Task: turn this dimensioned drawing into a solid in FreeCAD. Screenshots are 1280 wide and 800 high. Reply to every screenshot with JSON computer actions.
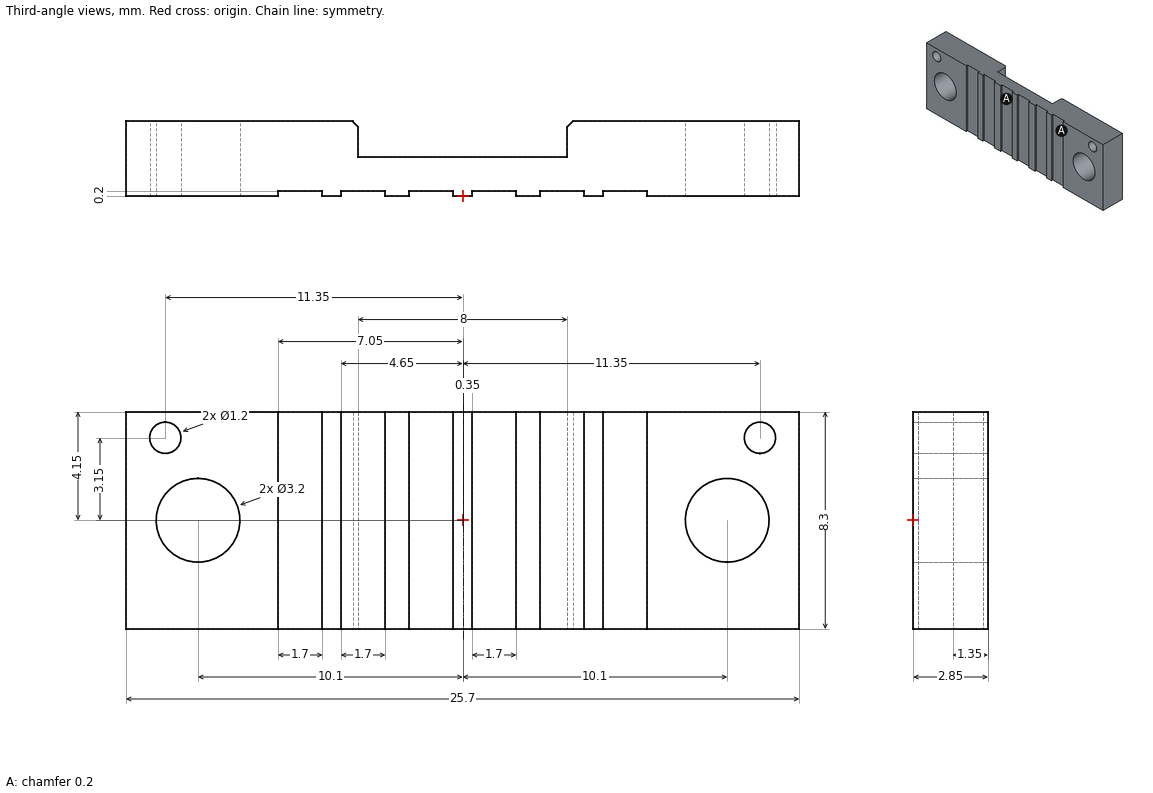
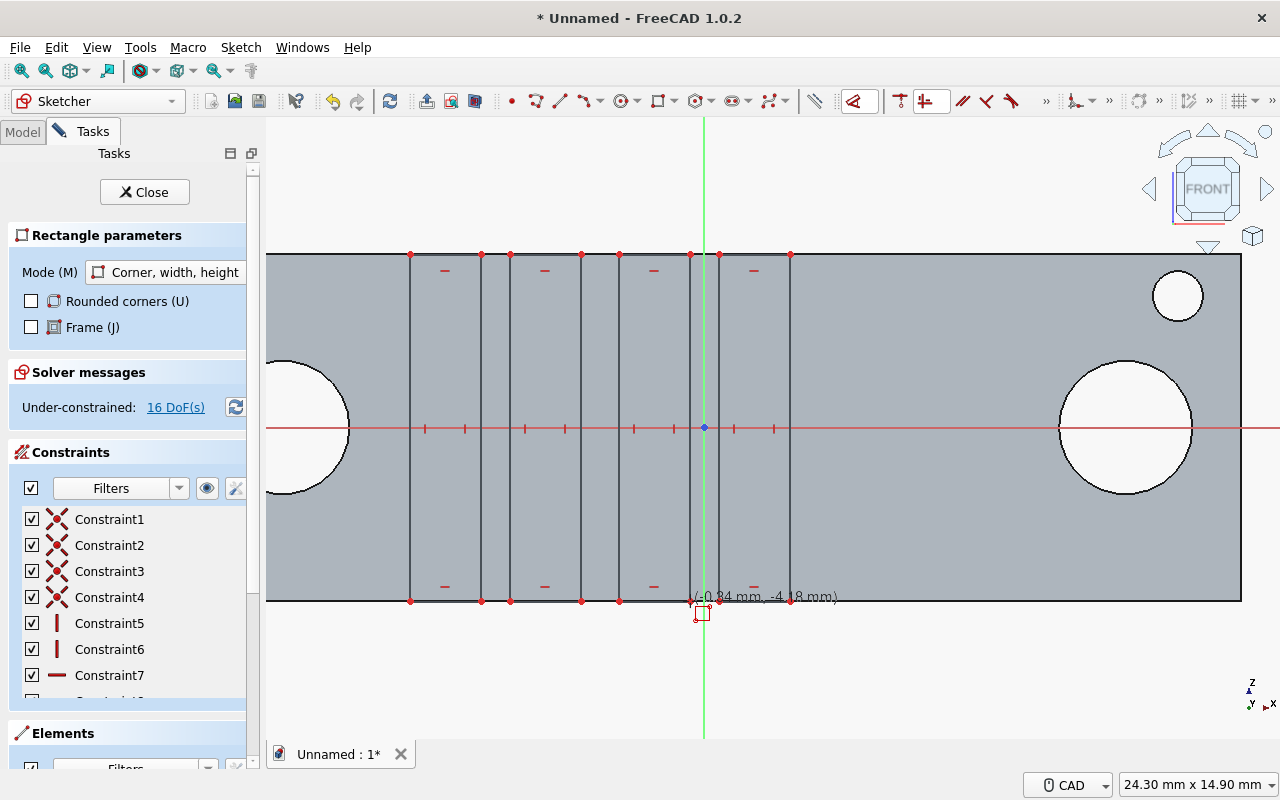
{"action": "left_click", "coordinate": [827, 254]}
{"action": "left_click", "coordinate": [898, 601]}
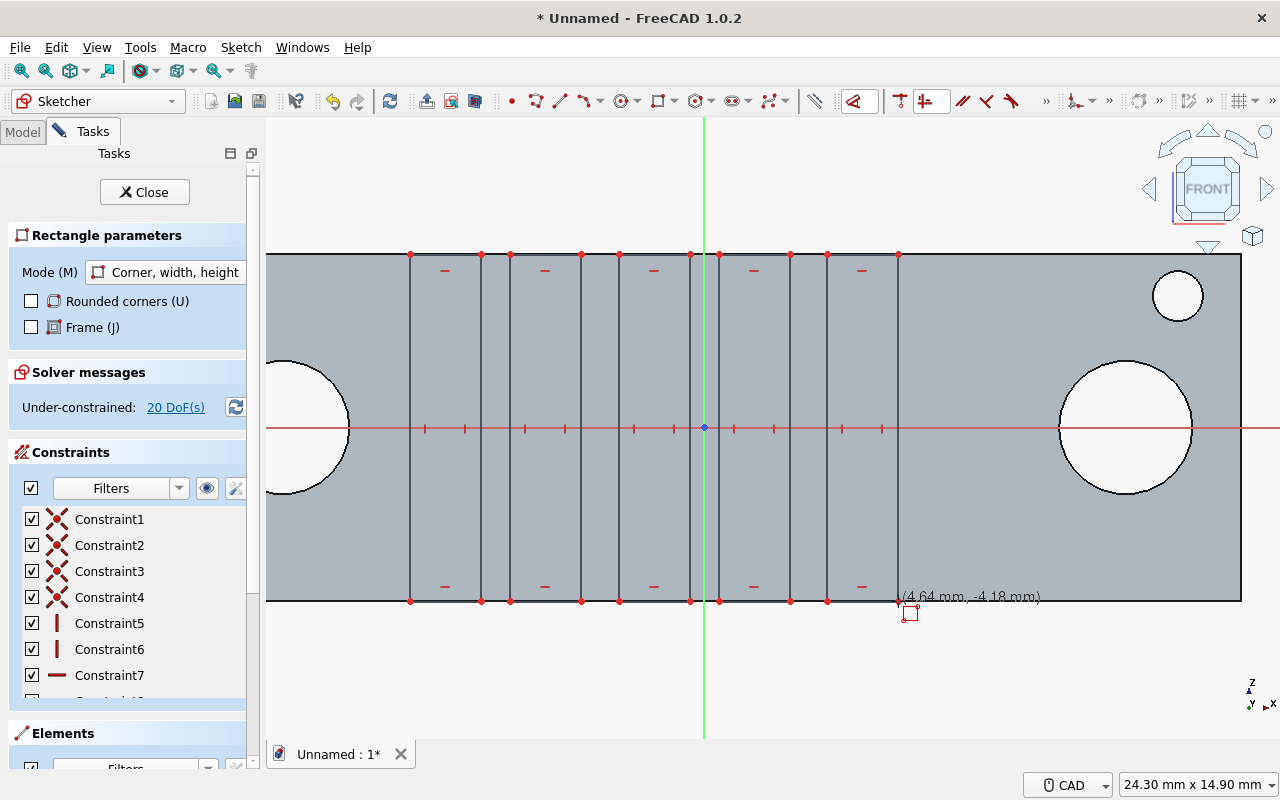
{"action": "left_click", "coordinate": [928, 254]}
{"action": "left_click", "coordinate": [999, 601]}
{"action": "key", "text": "Escape"}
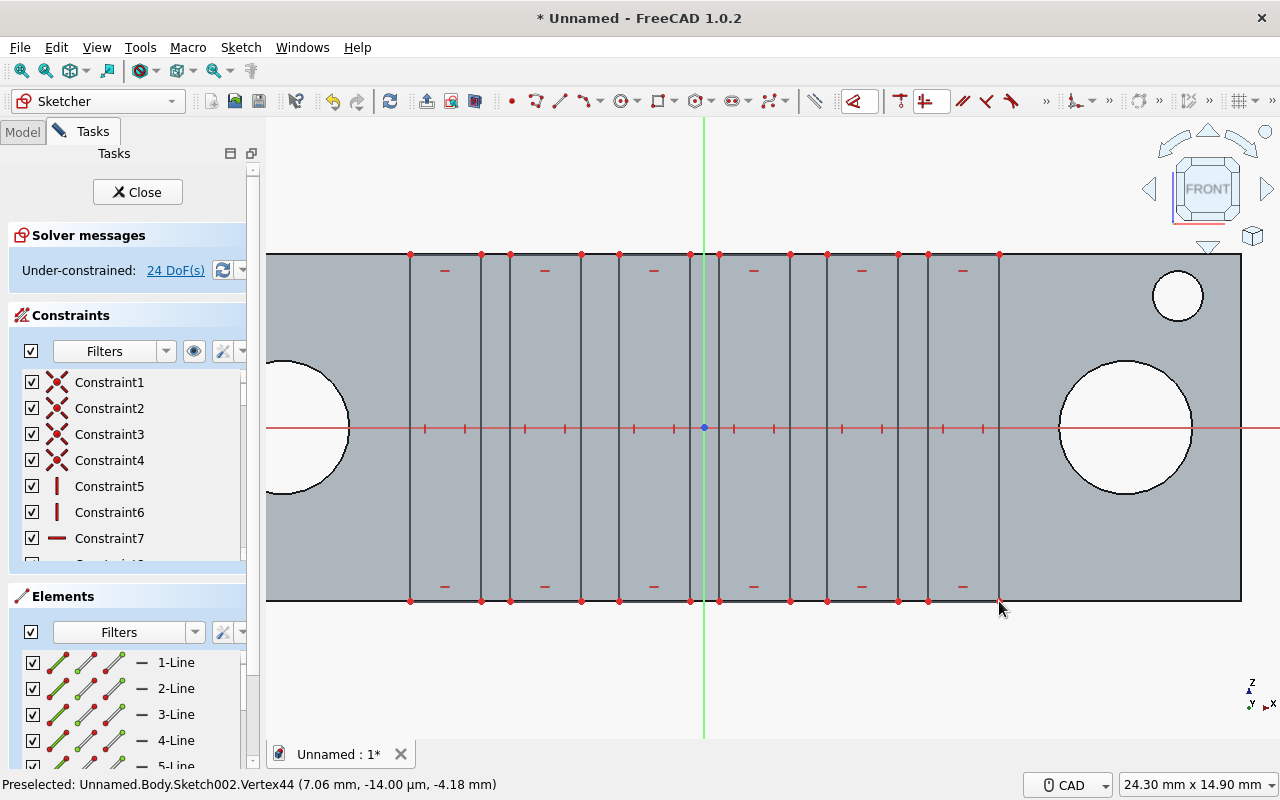
{"action": "left_click", "coordinate": [790, 255]}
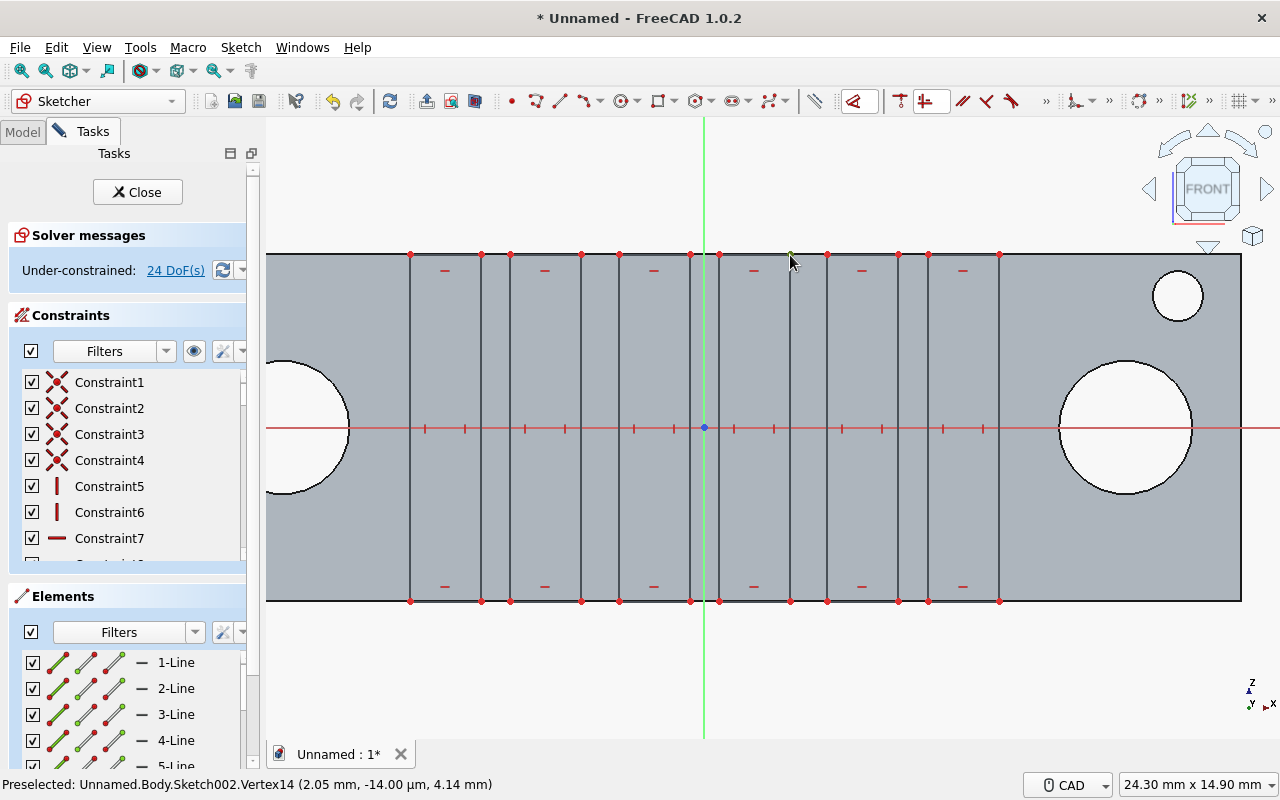
{"action": "left_click", "coordinate": [619, 255]}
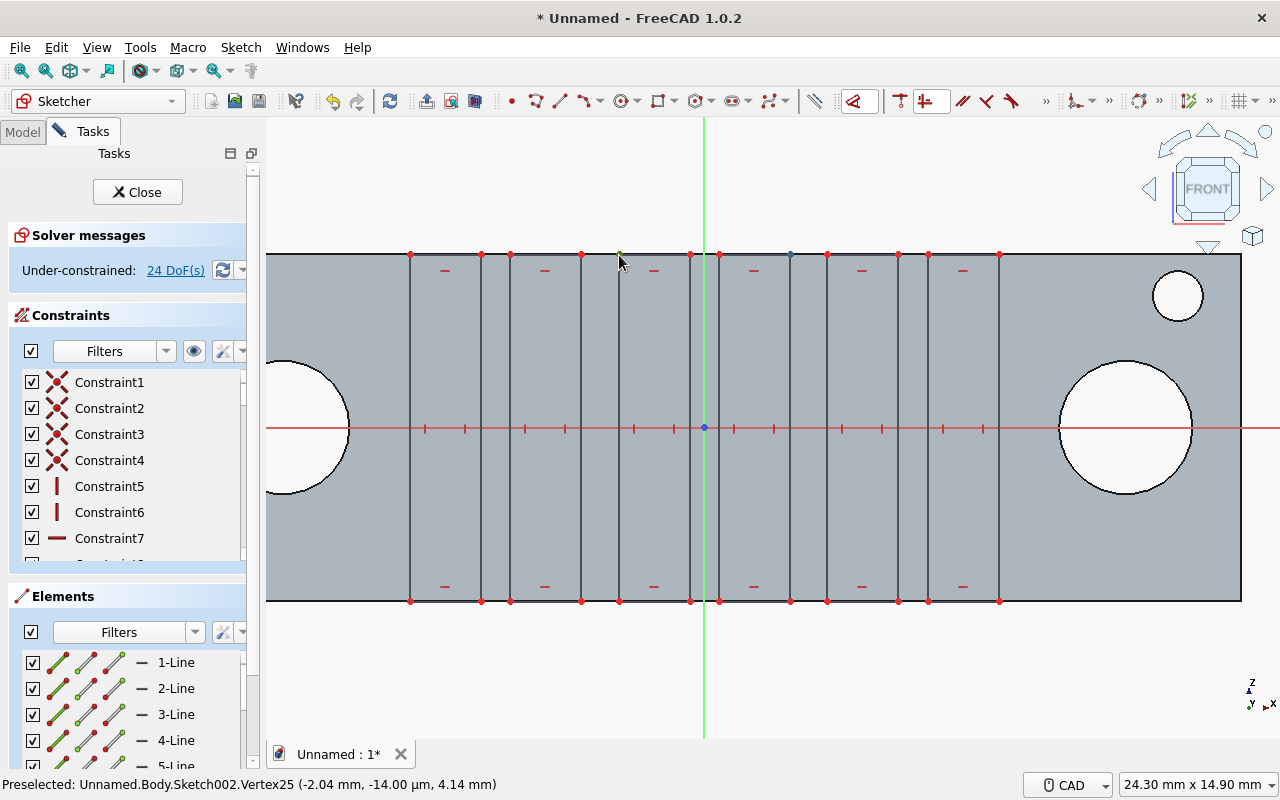
{"action": "left_click", "coordinate": [704, 671]}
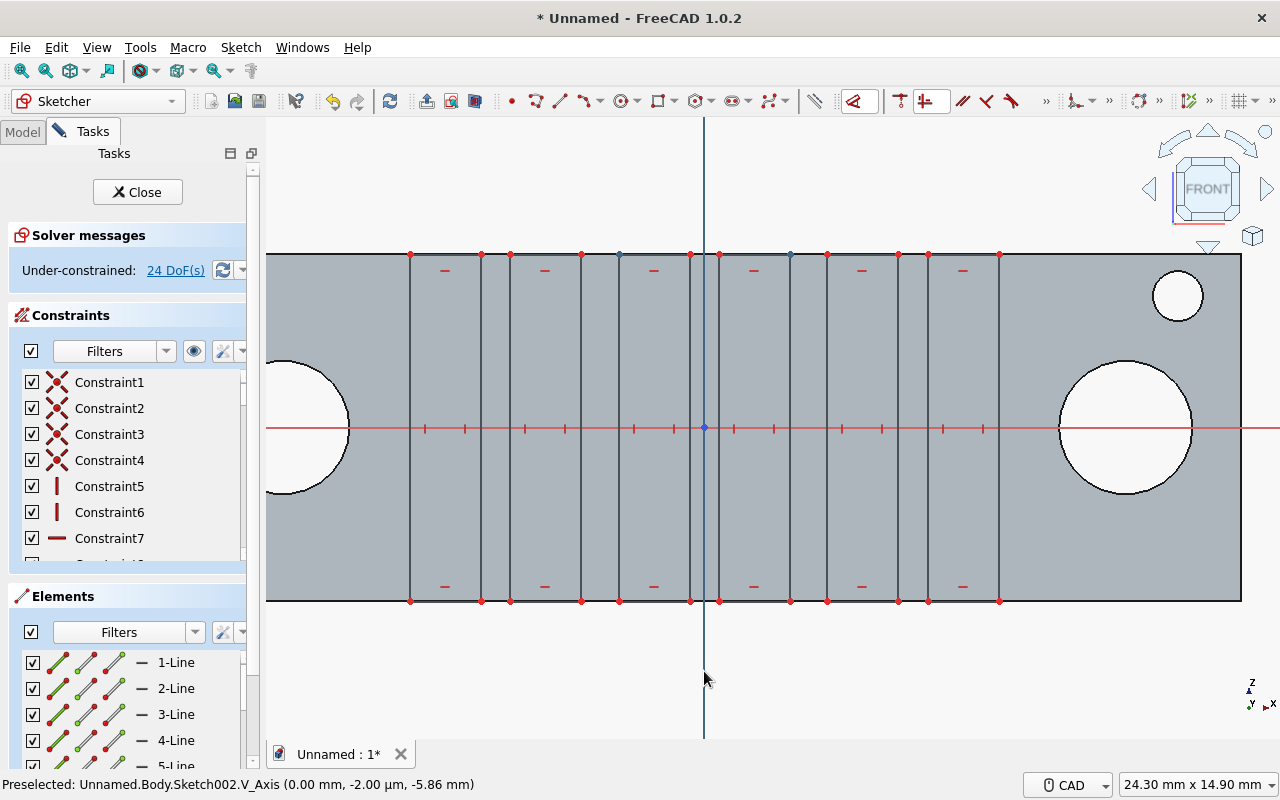
{"action": "key", "text": "s"}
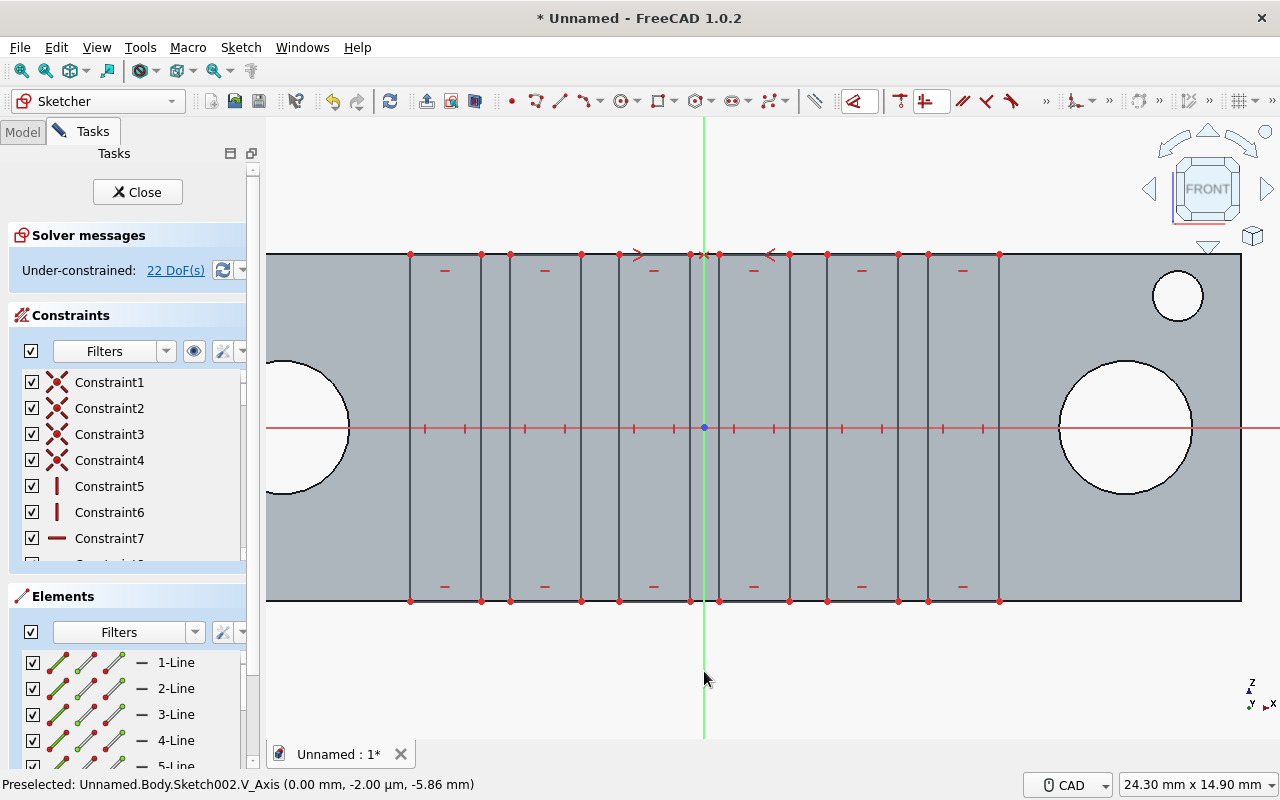
{"action": "left_click", "coordinate": [719, 602]}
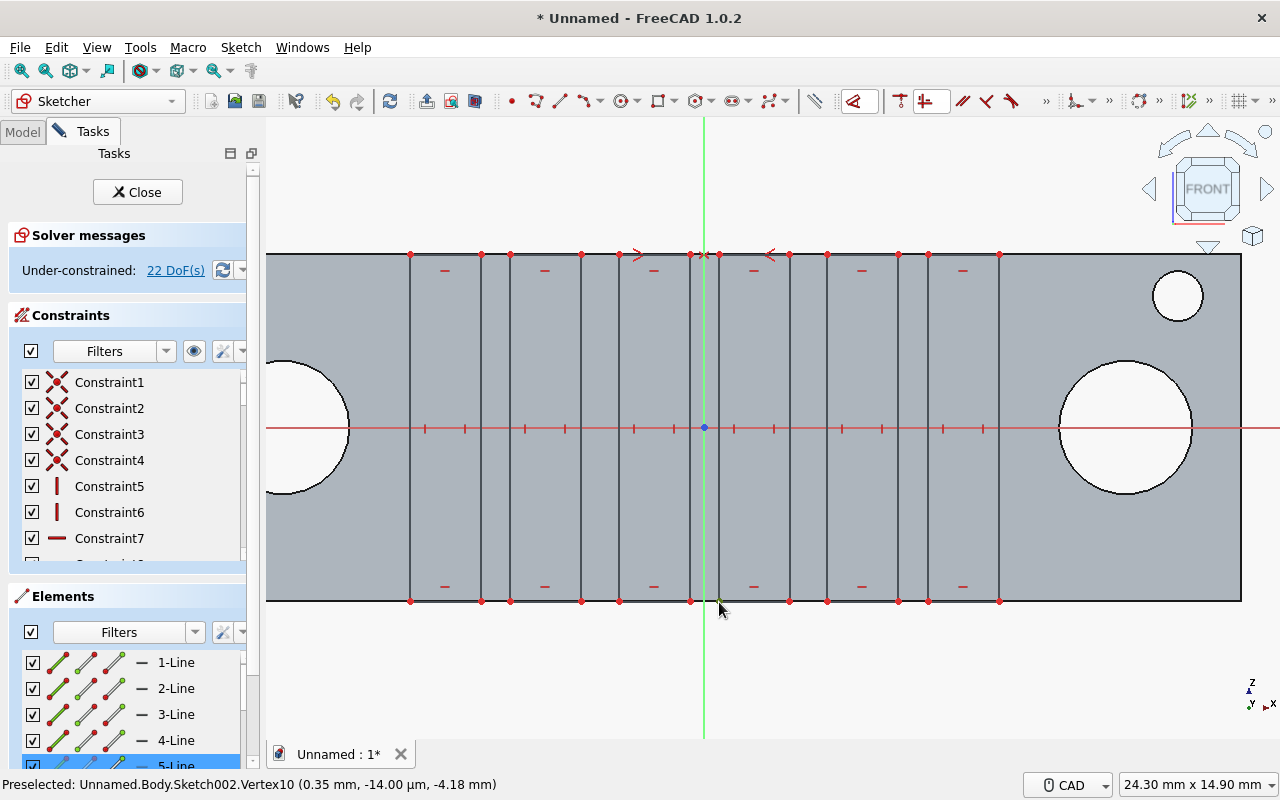
{"action": "left_click", "coordinate": [690, 602]}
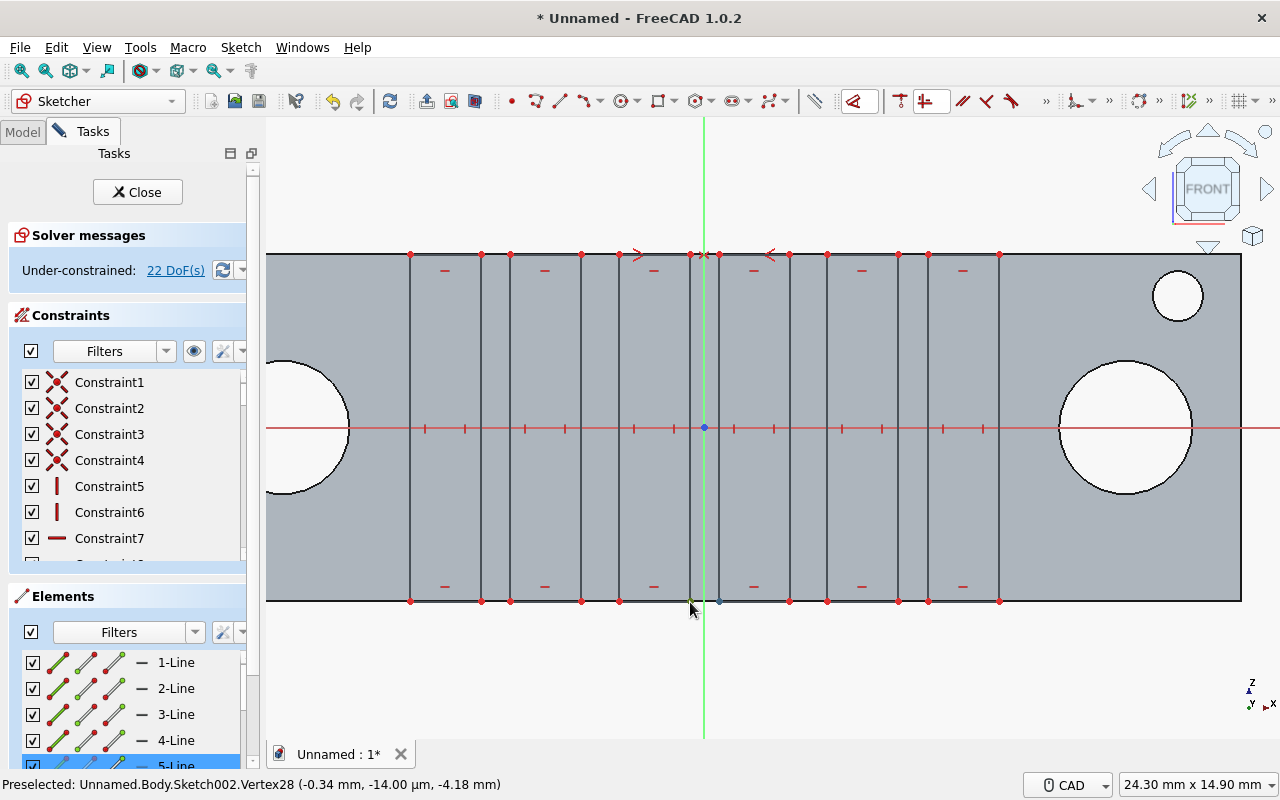
{"action": "left_click", "coordinate": [704, 671]}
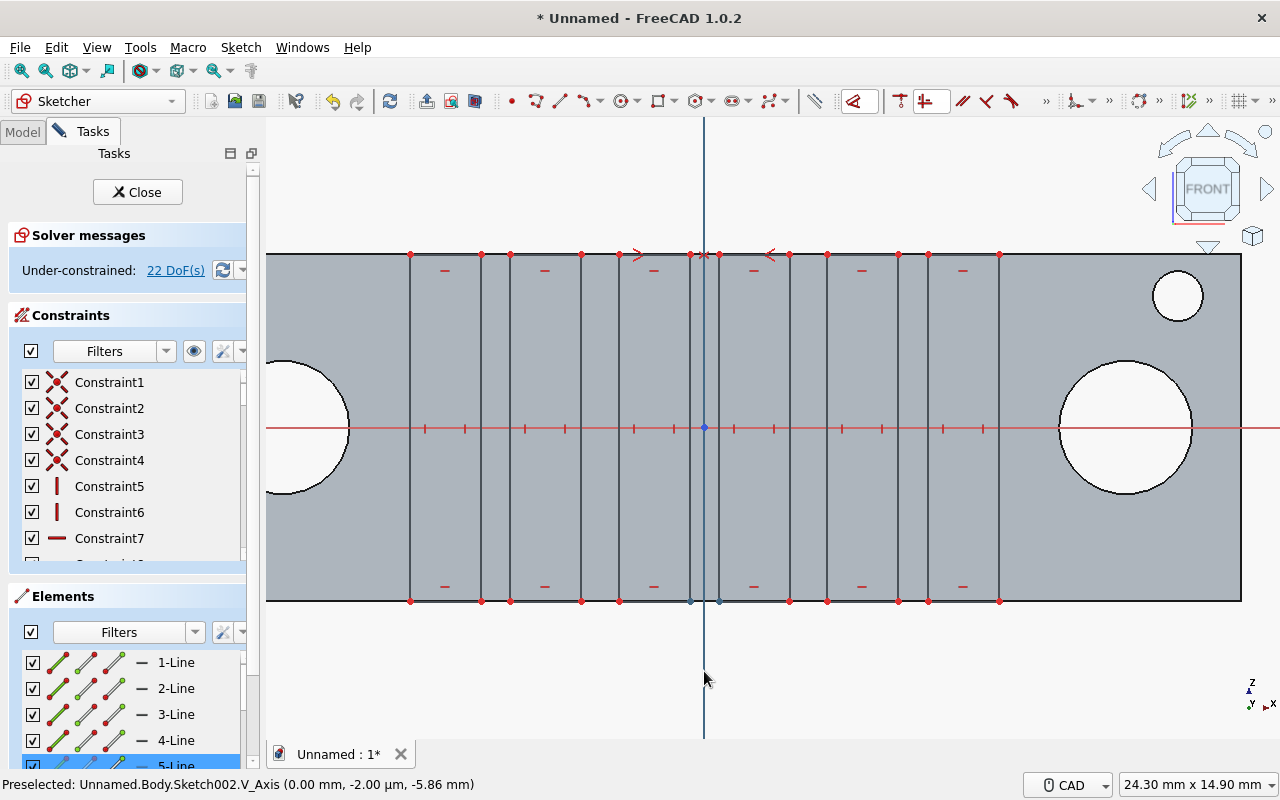
{"action": "key", "text": "s"}